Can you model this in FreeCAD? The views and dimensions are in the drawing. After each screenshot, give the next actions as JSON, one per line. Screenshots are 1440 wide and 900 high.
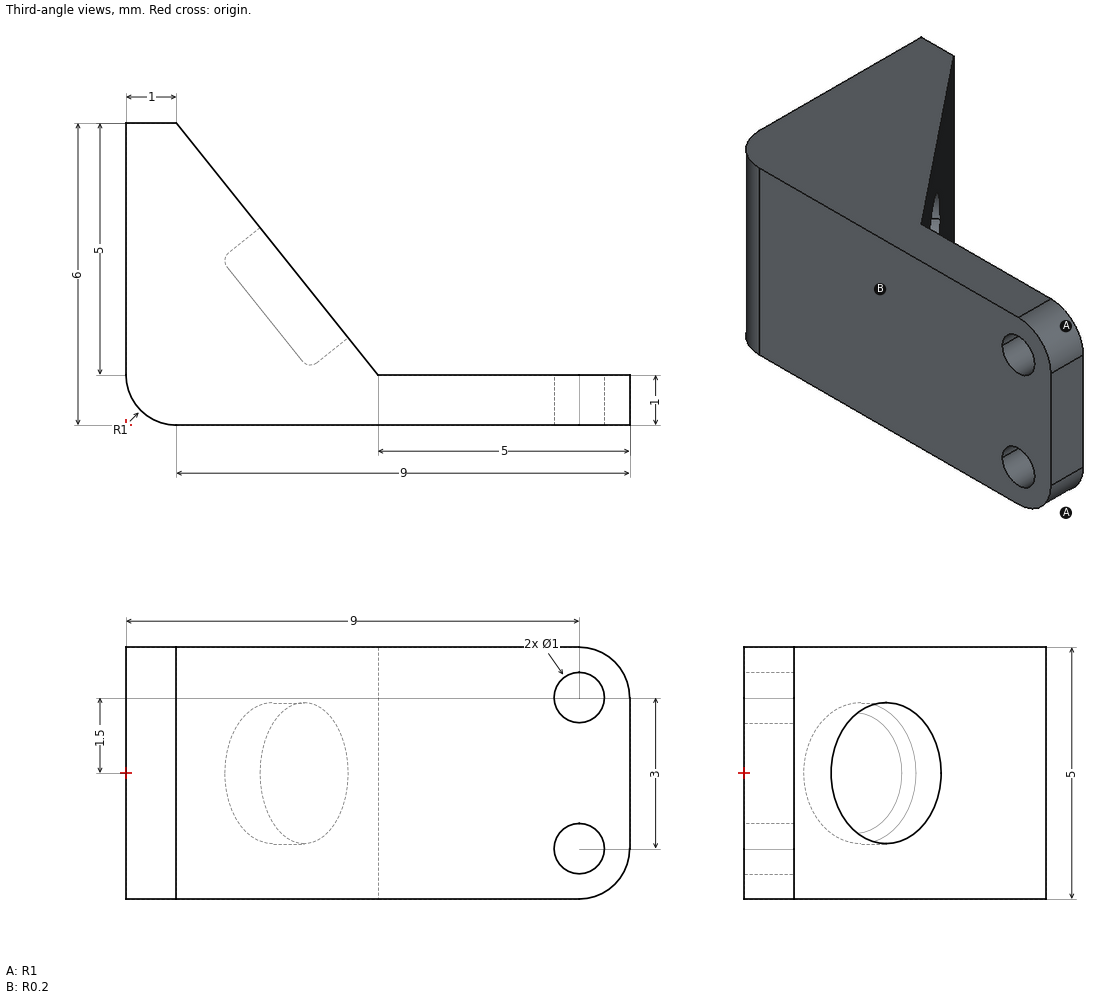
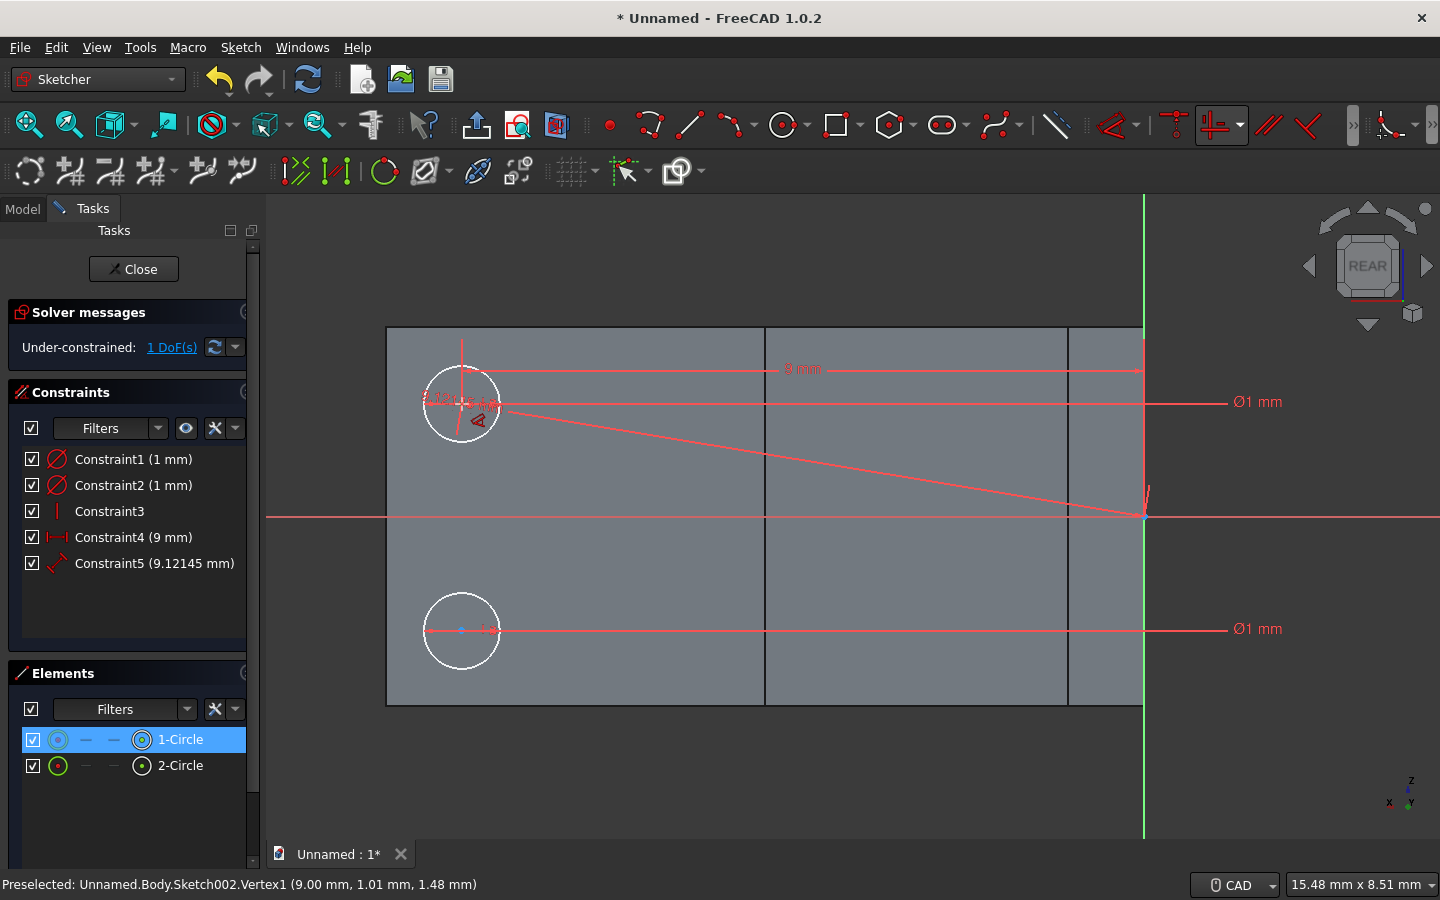
{"action": "left_click", "coordinate": [462, 631]}
{"action": "left_click", "coordinate": [428, 465]}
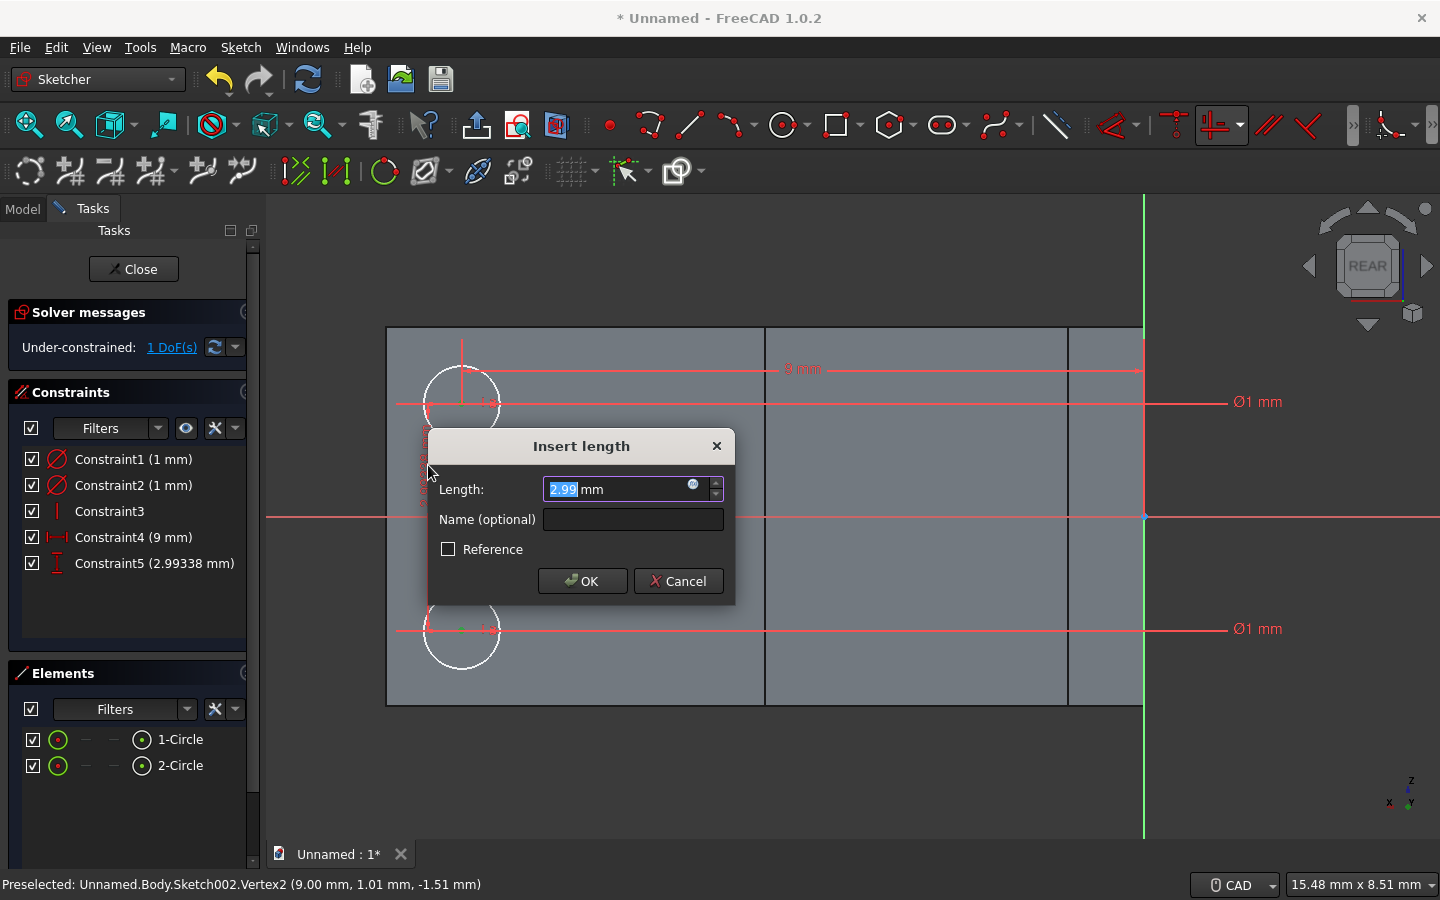
{"action": "type", "text": "3"}
{"action": "key", "text": "Return"}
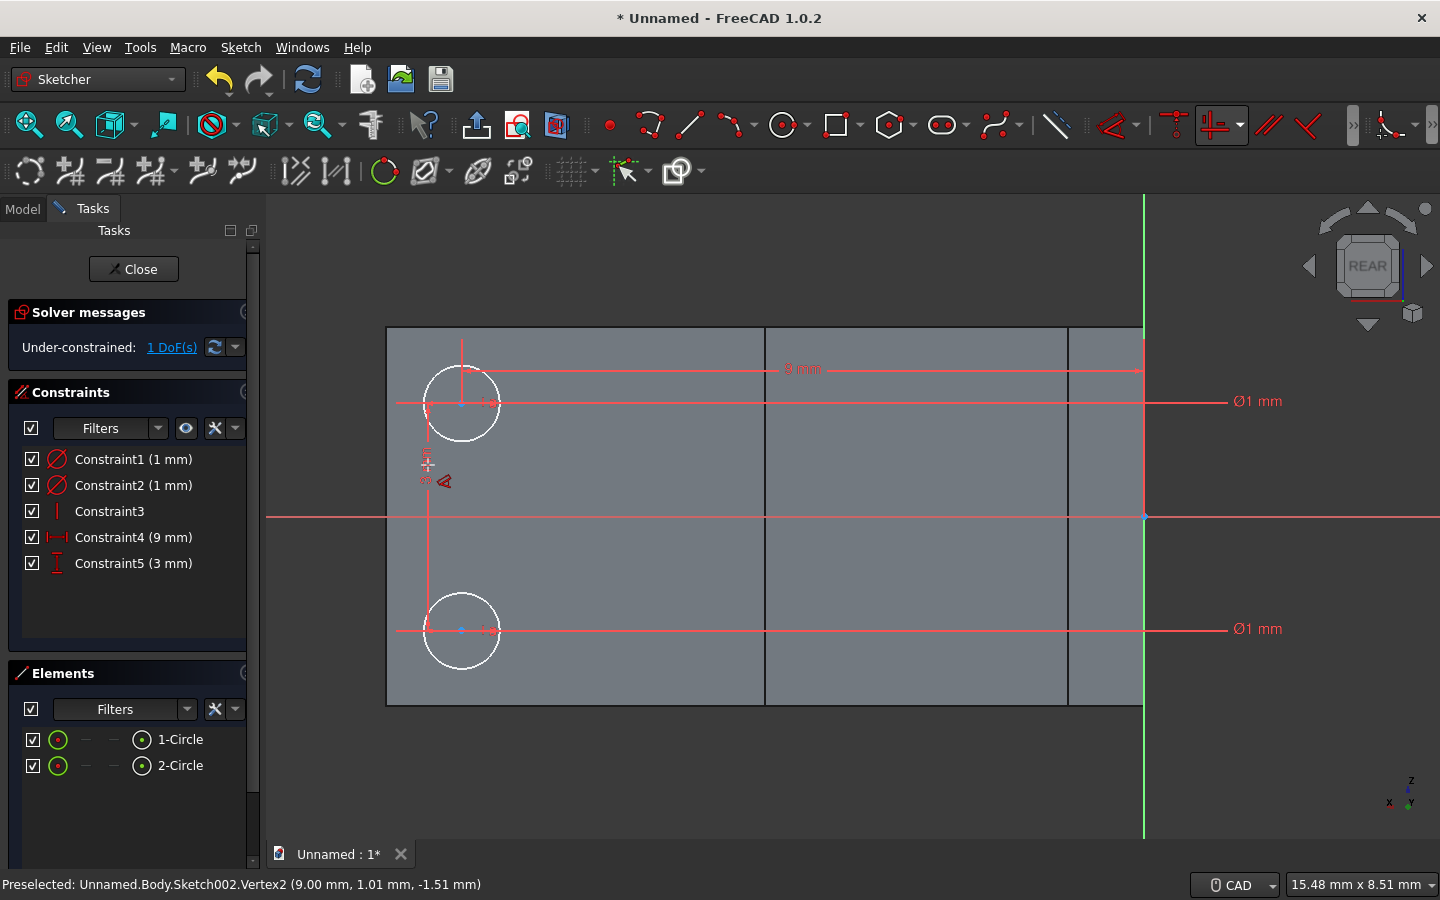
{"action": "left_click", "coordinate": [462, 403]}
{"action": "left_click", "coordinate": [1178, 460]}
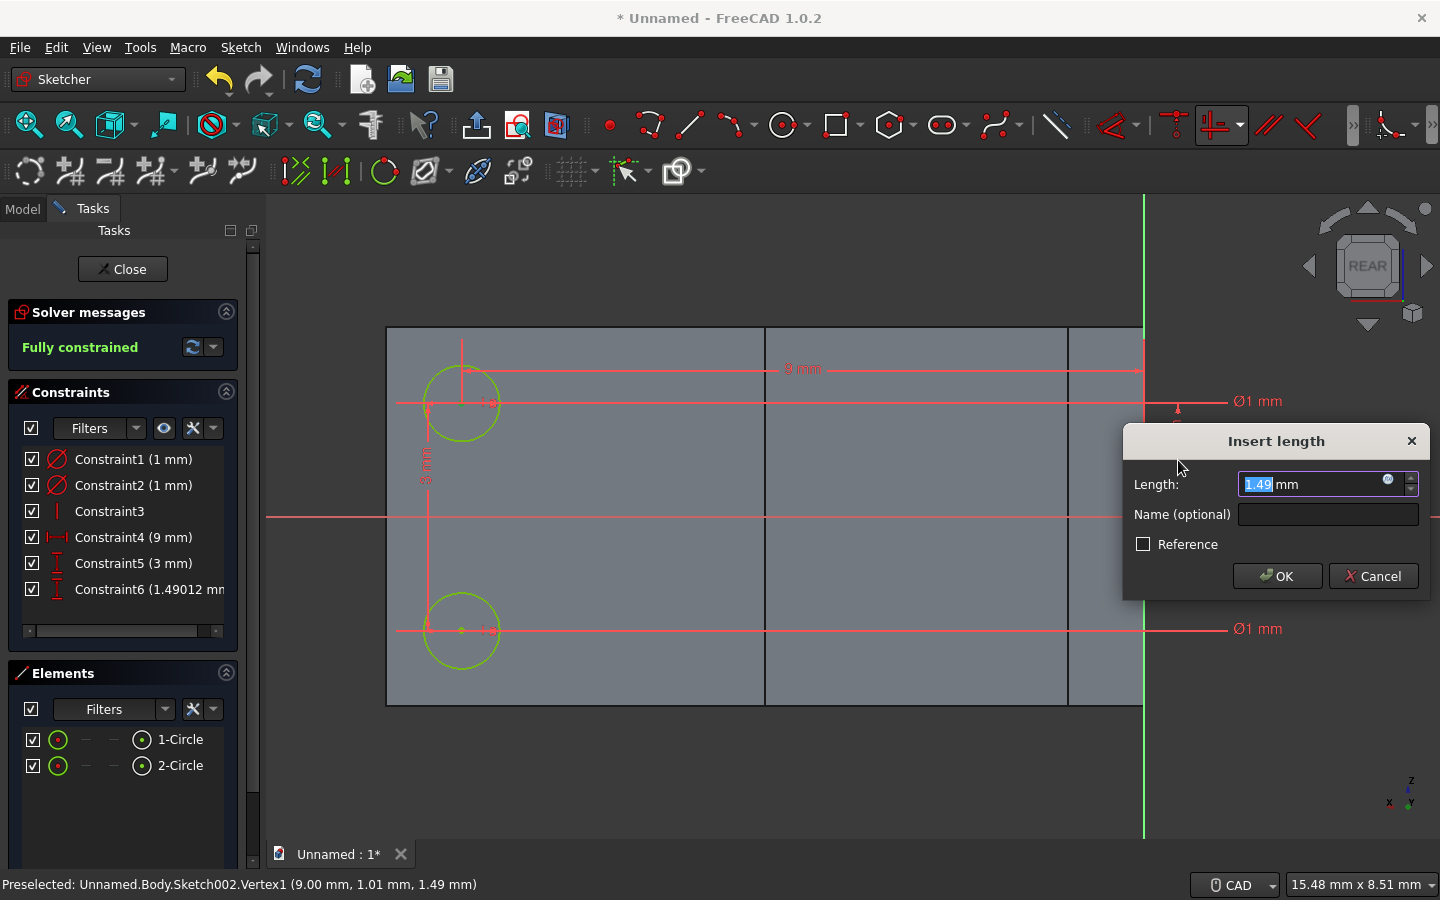
{"action": "type", "text": "1.5"}
{"action": "key", "text": "Return"}
{"action": "key", "text": "Escape"}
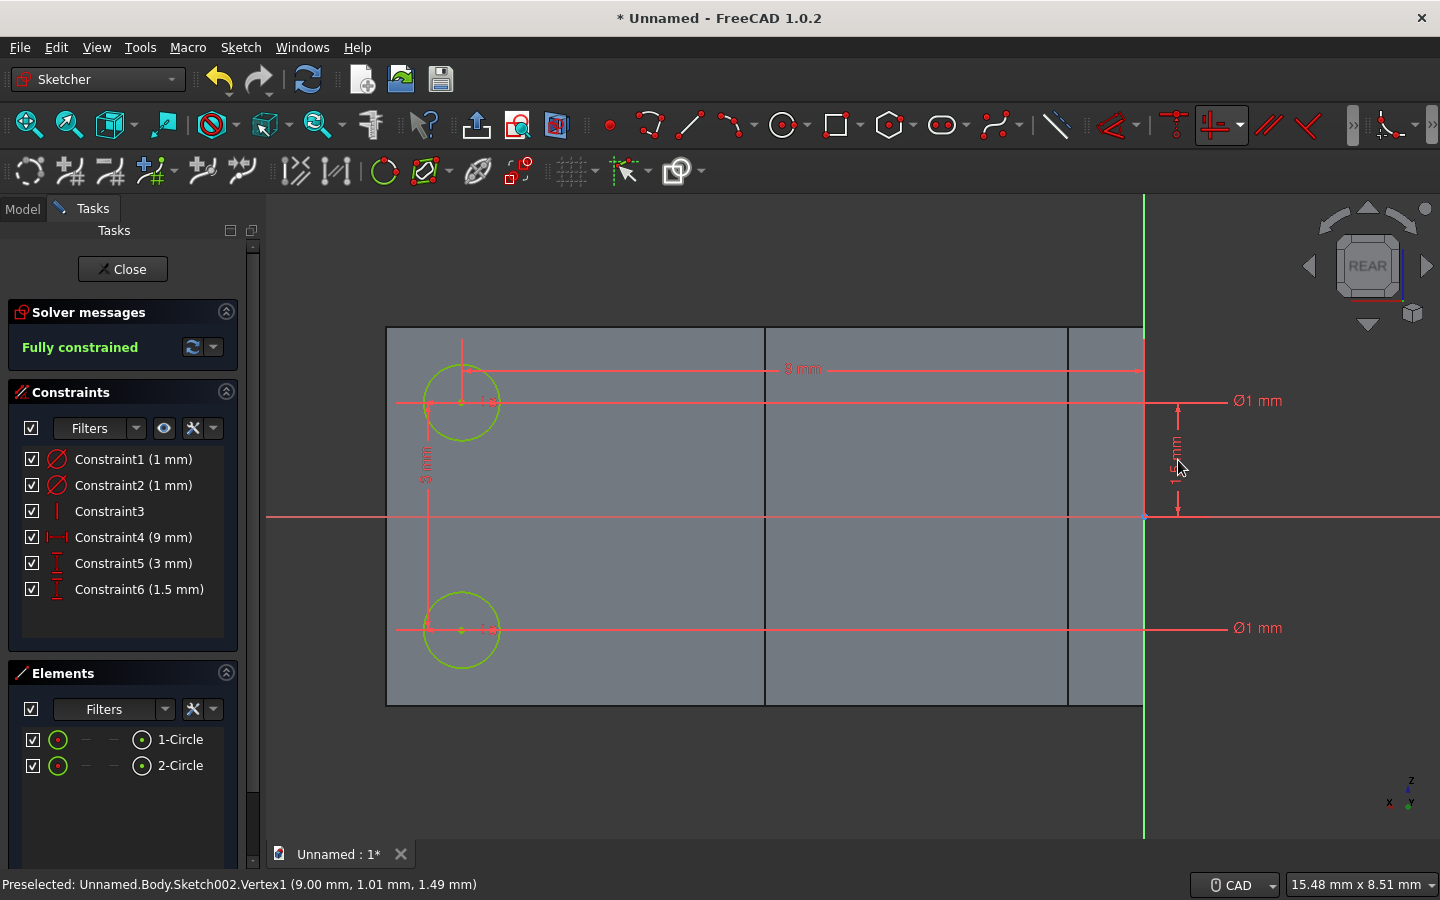
{"action": "left_click", "coordinate": [123, 269]}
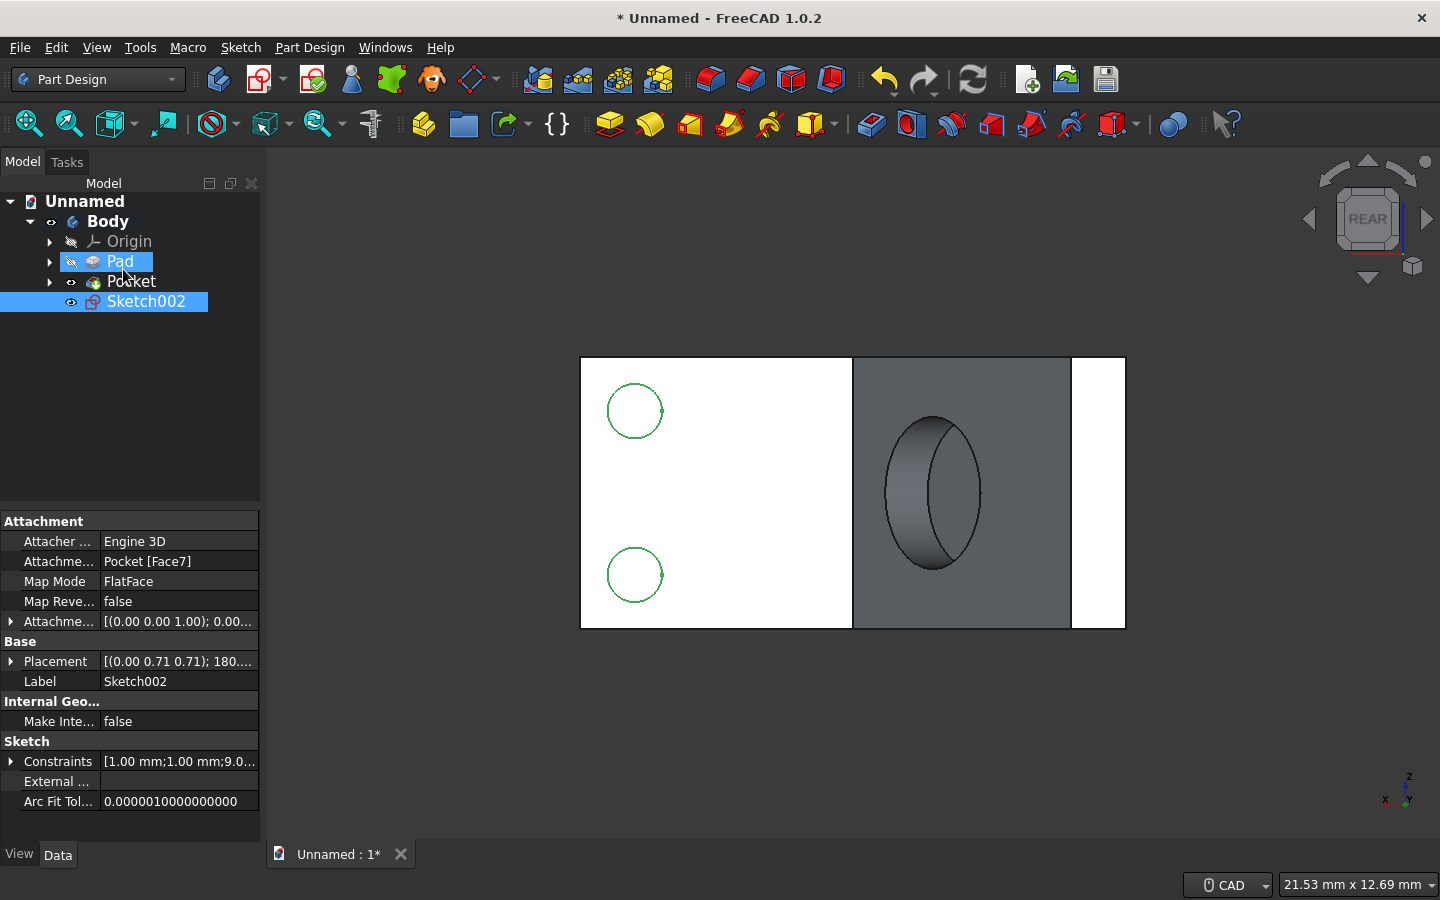
{"action": "left_click", "coordinate": [872, 124]}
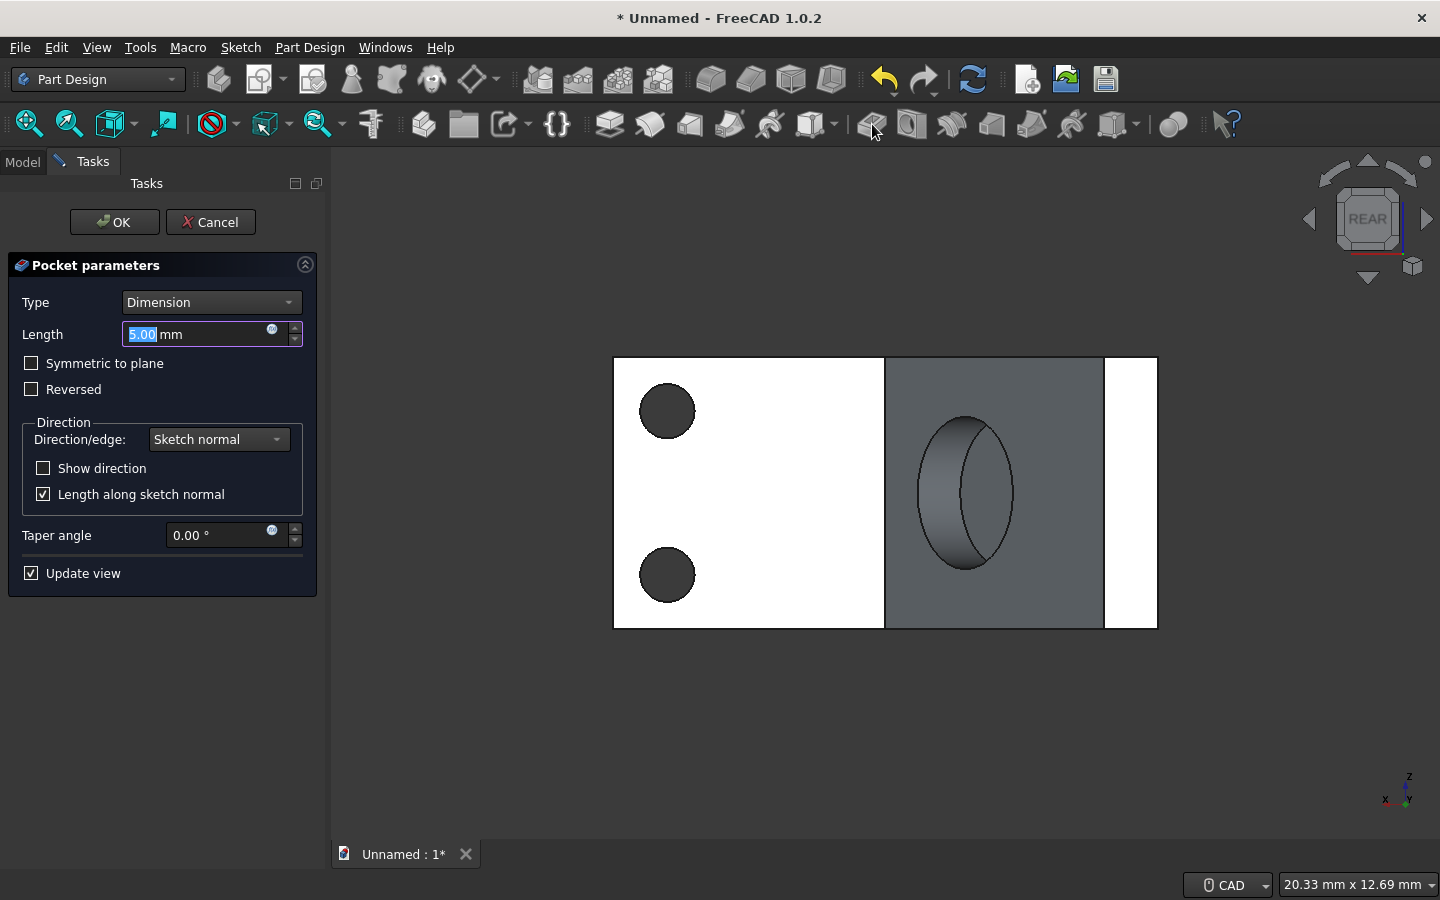
{"action": "left_click", "coordinate": [212, 302]}